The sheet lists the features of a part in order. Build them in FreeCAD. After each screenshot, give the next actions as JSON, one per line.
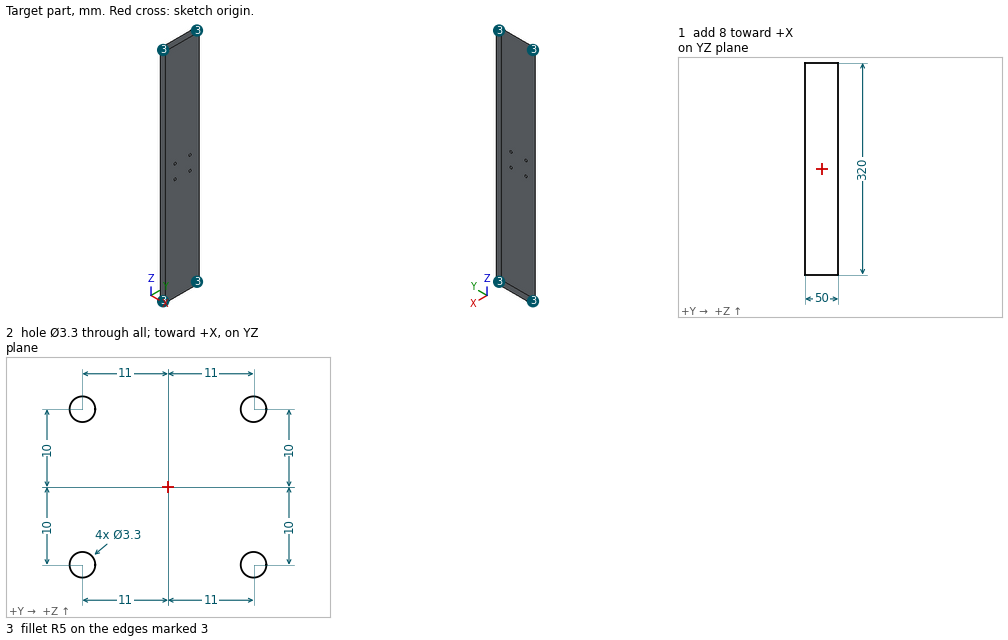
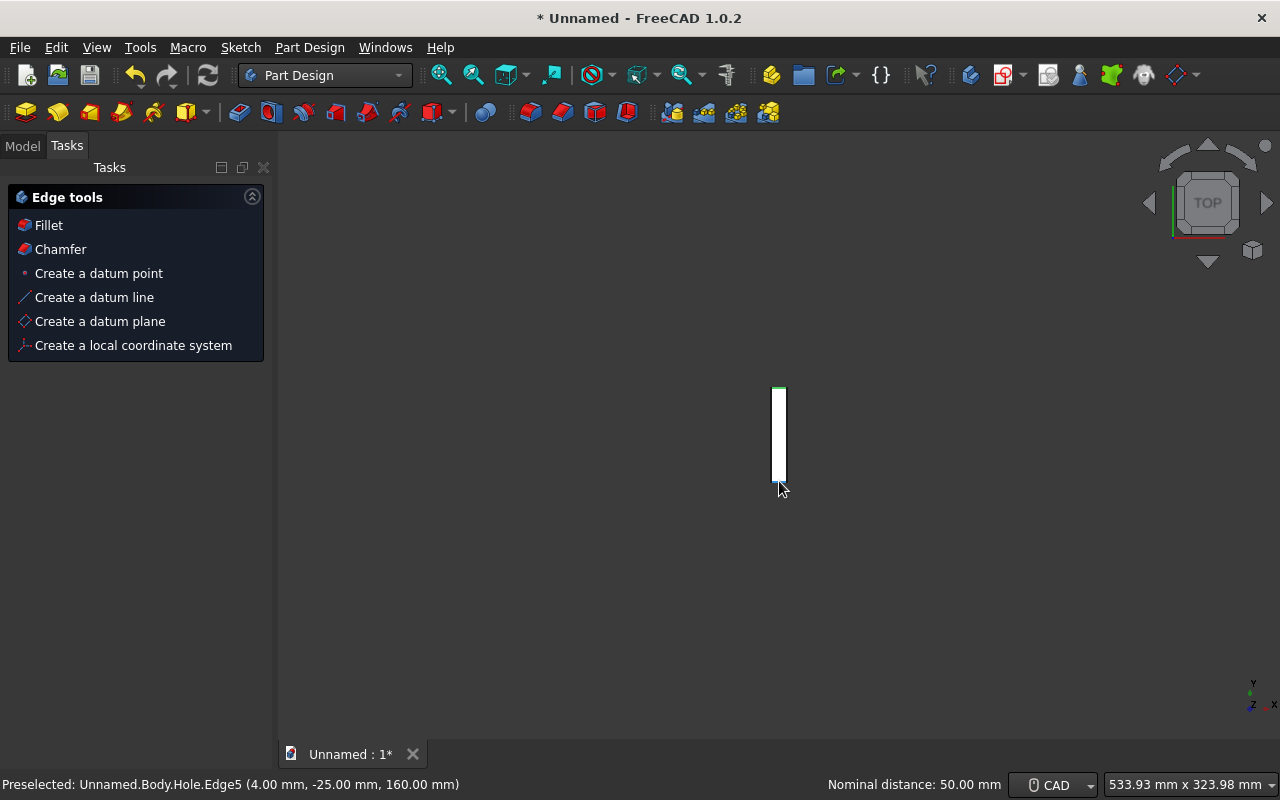
{"action": "key", "text": "1"}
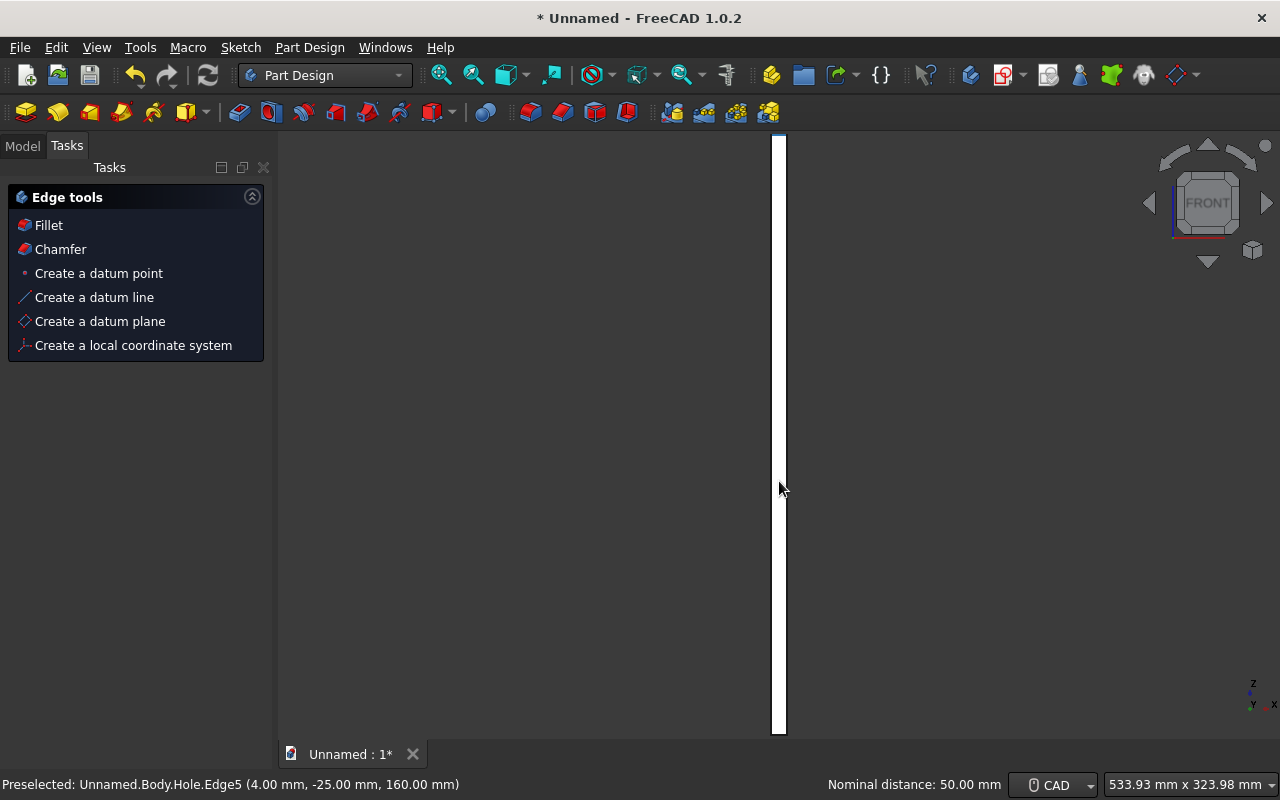
{"action": "key", "text": "3"}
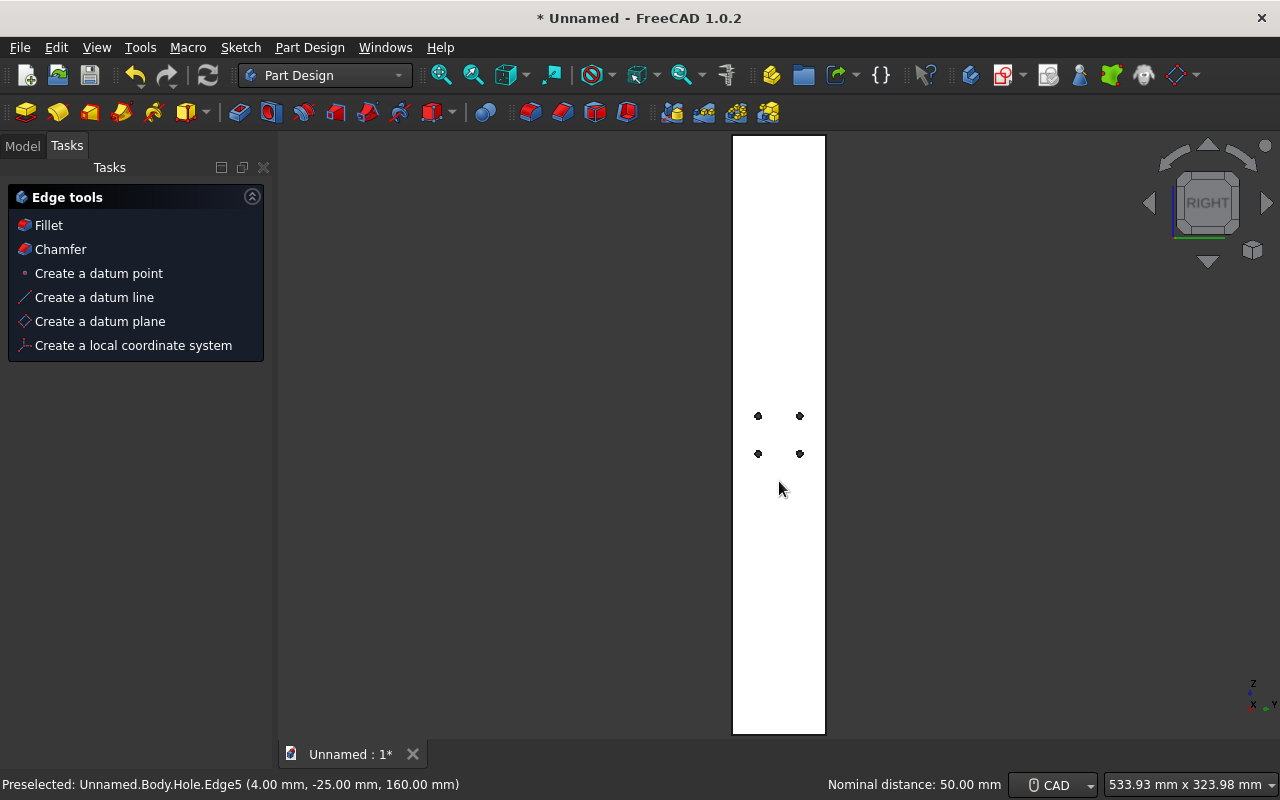
{"action": "key", "text": "5"}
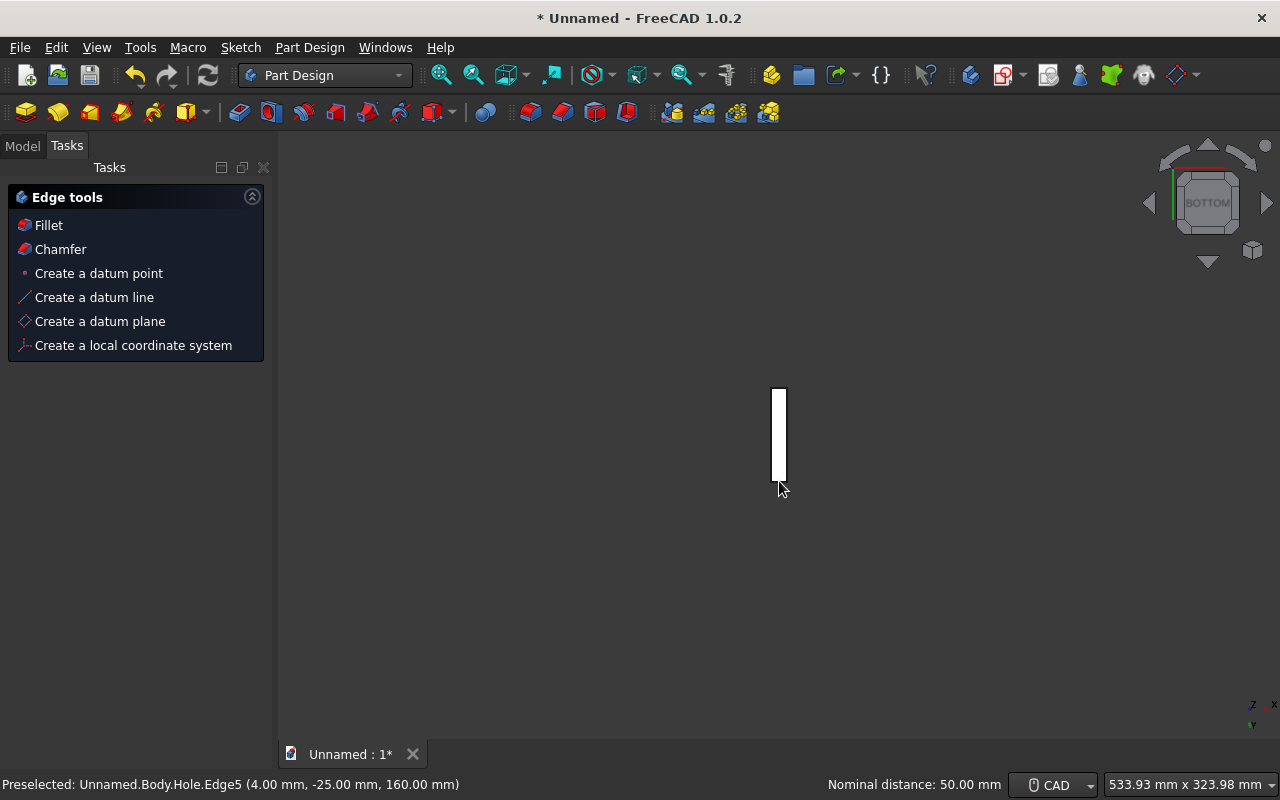
{"action": "left_click", "coordinate": [442, 76]}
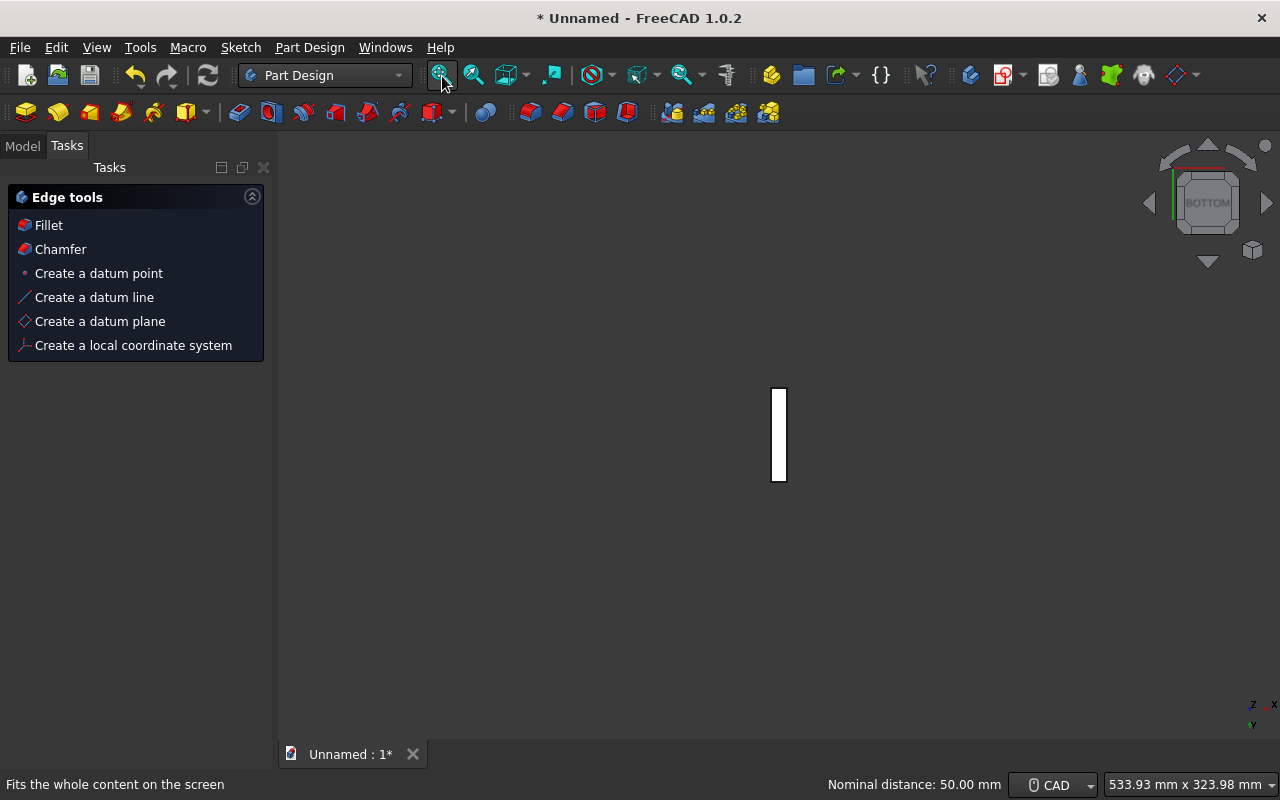
{"action": "left_click", "coordinate": [779, 387], "text": "ctrl"}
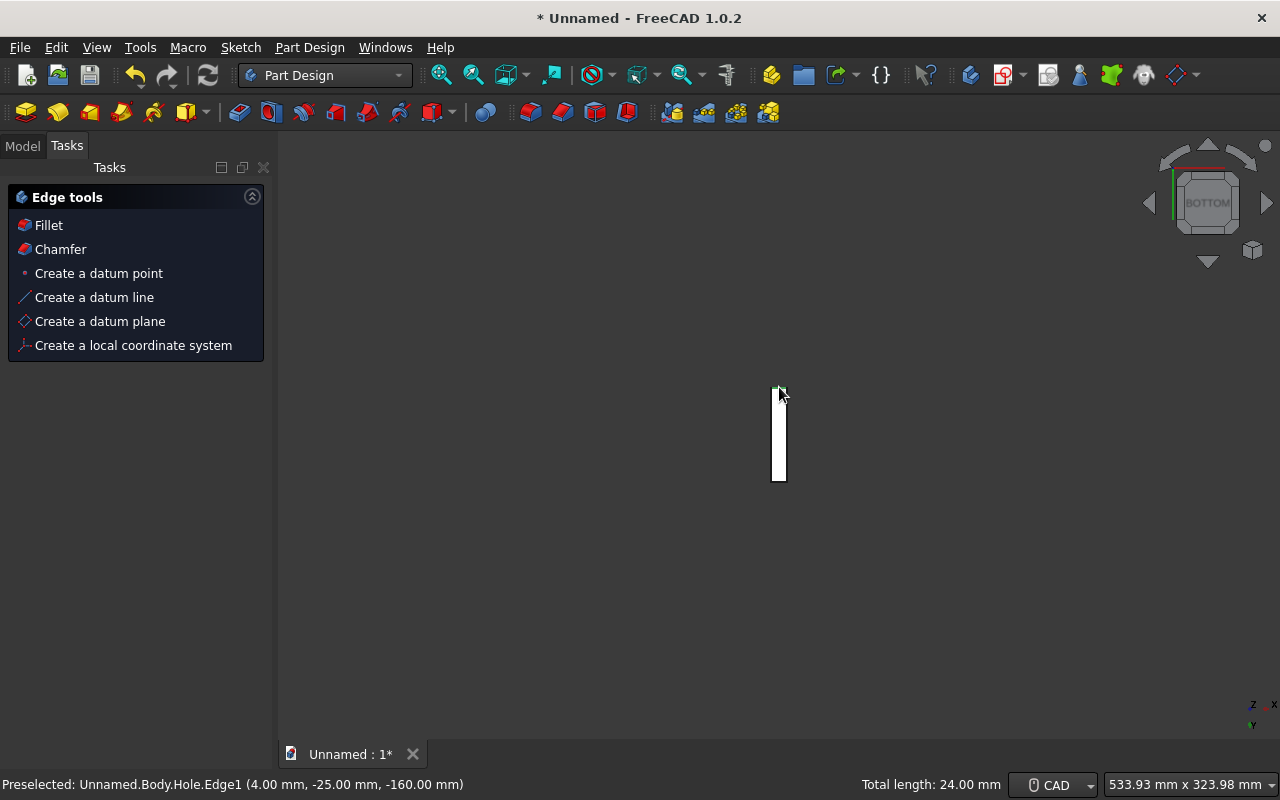
{"action": "left_click", "coordinate": [779, 481], "text": "ctrl"}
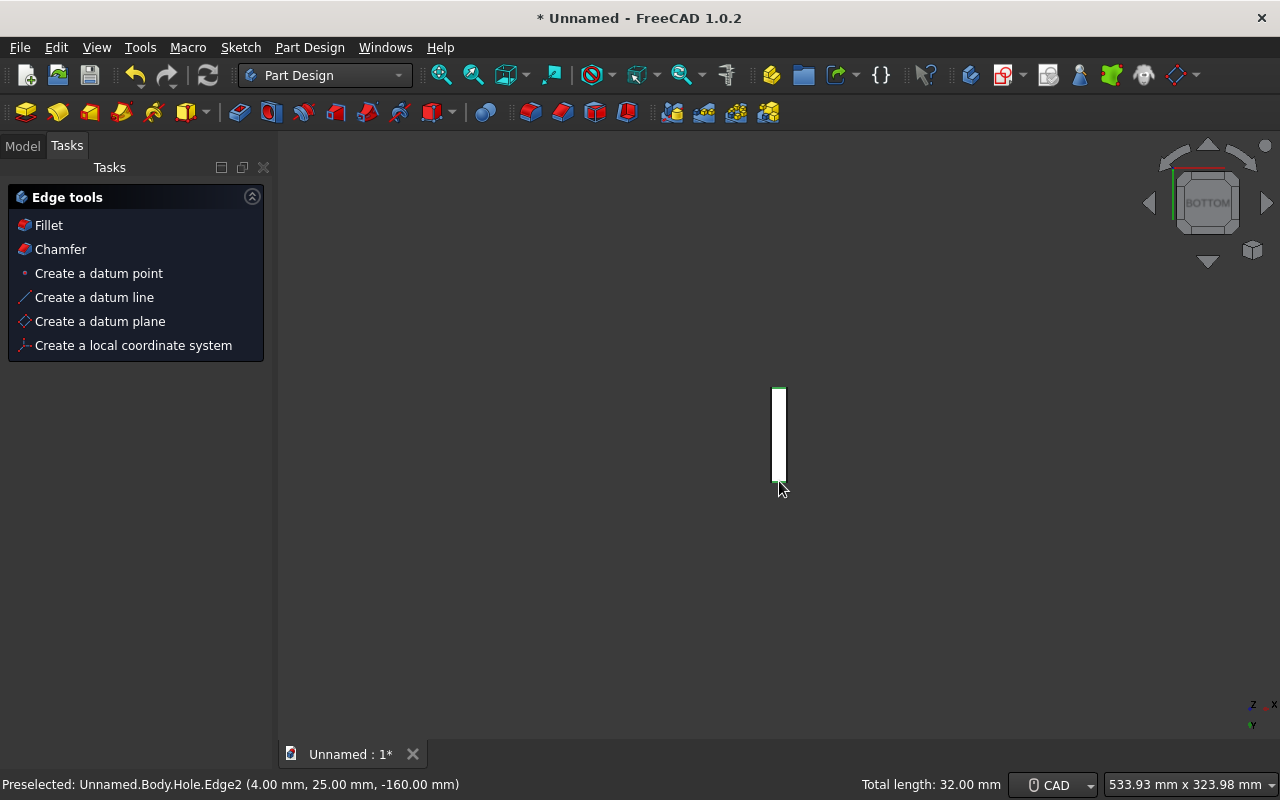
{"action": "left_click", "coordinate": [532, 112]}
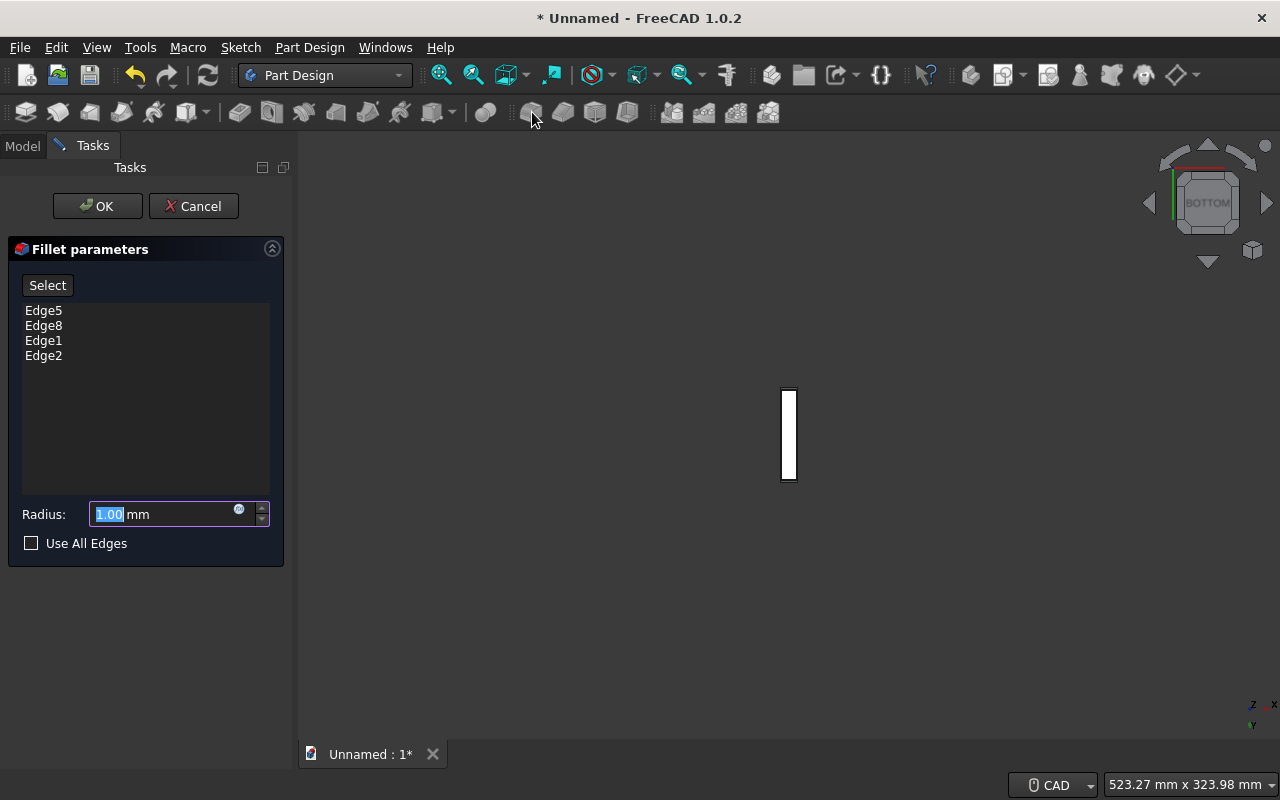
{"action": "type", "text": "5"}
{"action": "key", "text": "Tab"}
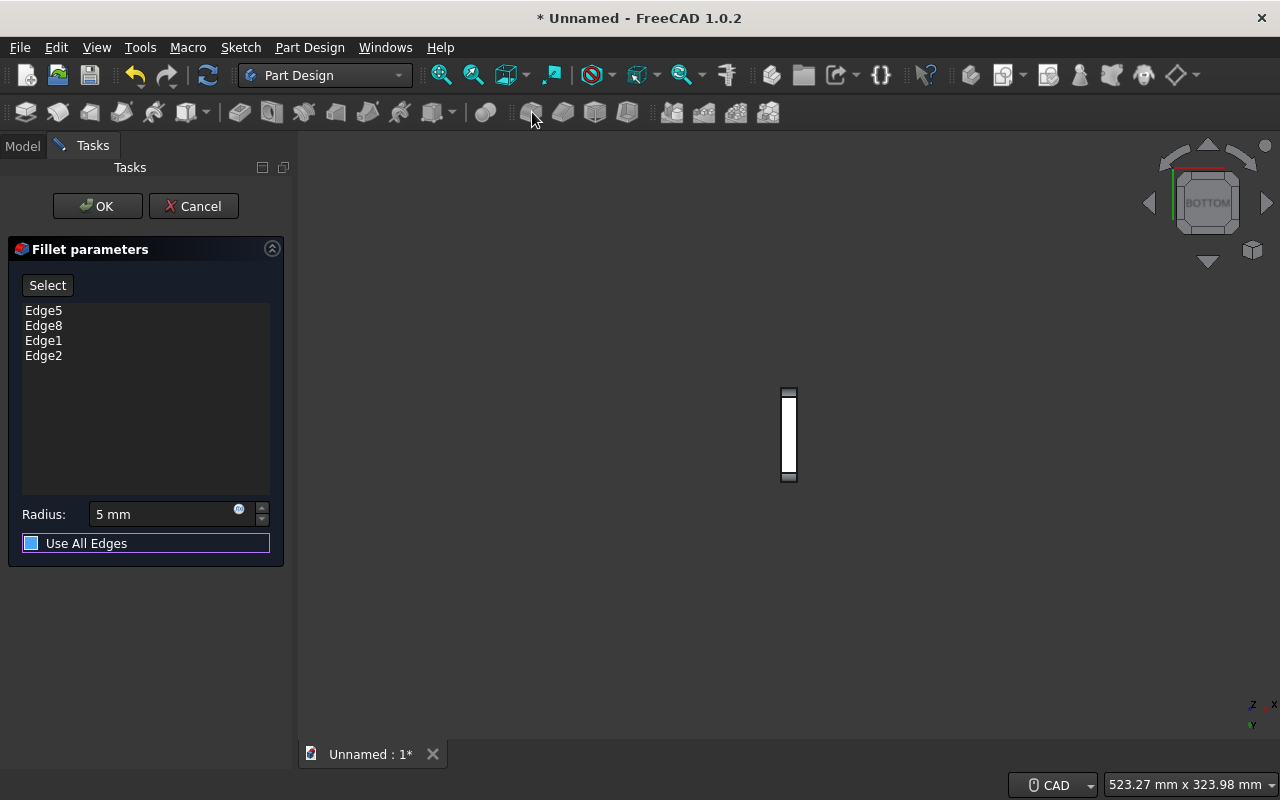
{"action": "left_click", "coordinate": [98, 206]}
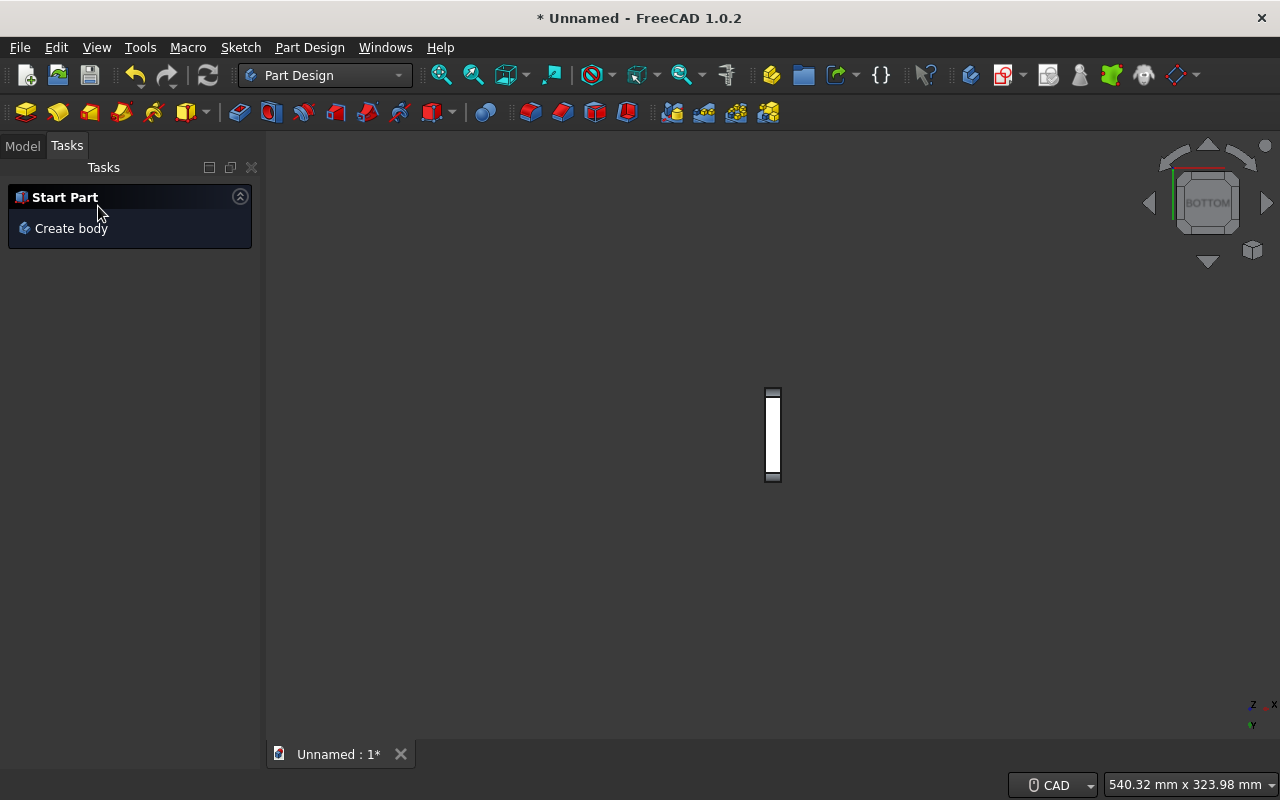
{"action": "key", "text": "0"}